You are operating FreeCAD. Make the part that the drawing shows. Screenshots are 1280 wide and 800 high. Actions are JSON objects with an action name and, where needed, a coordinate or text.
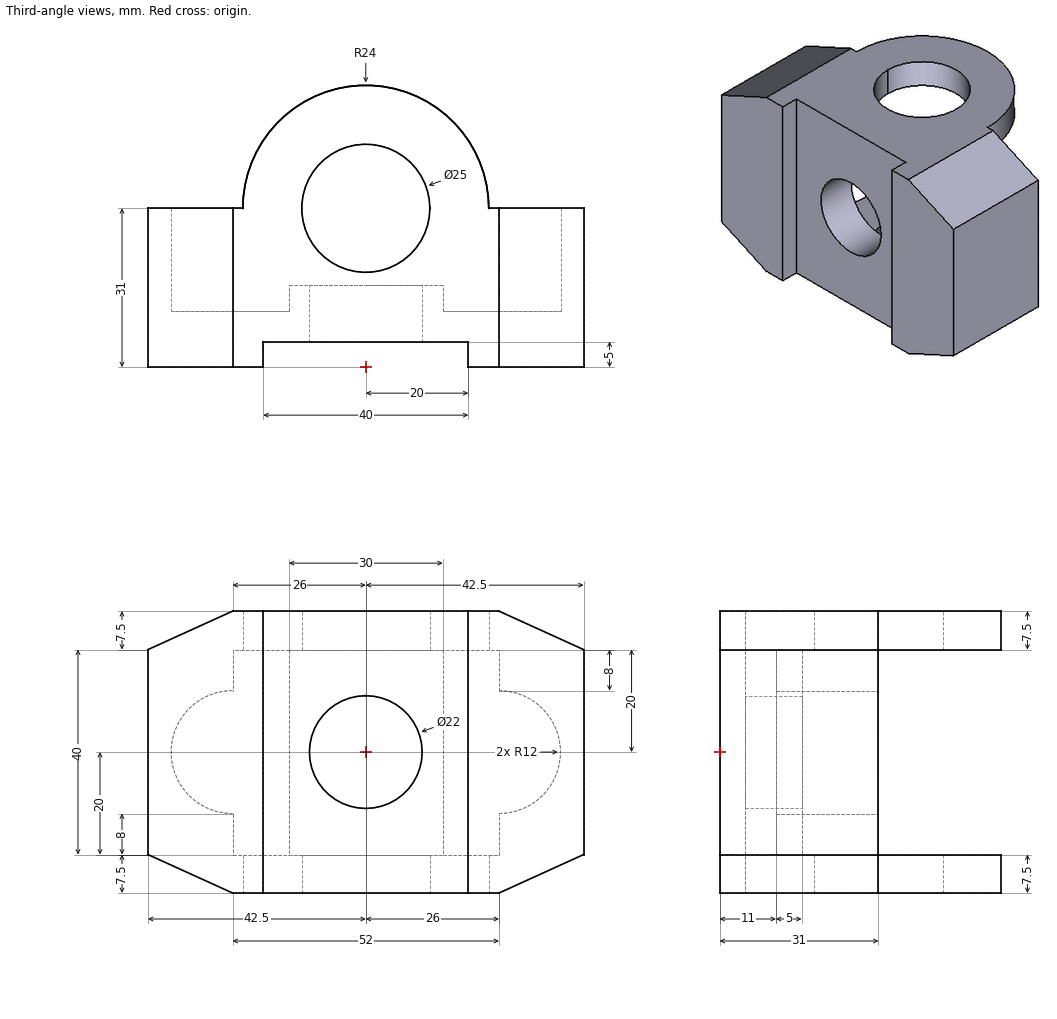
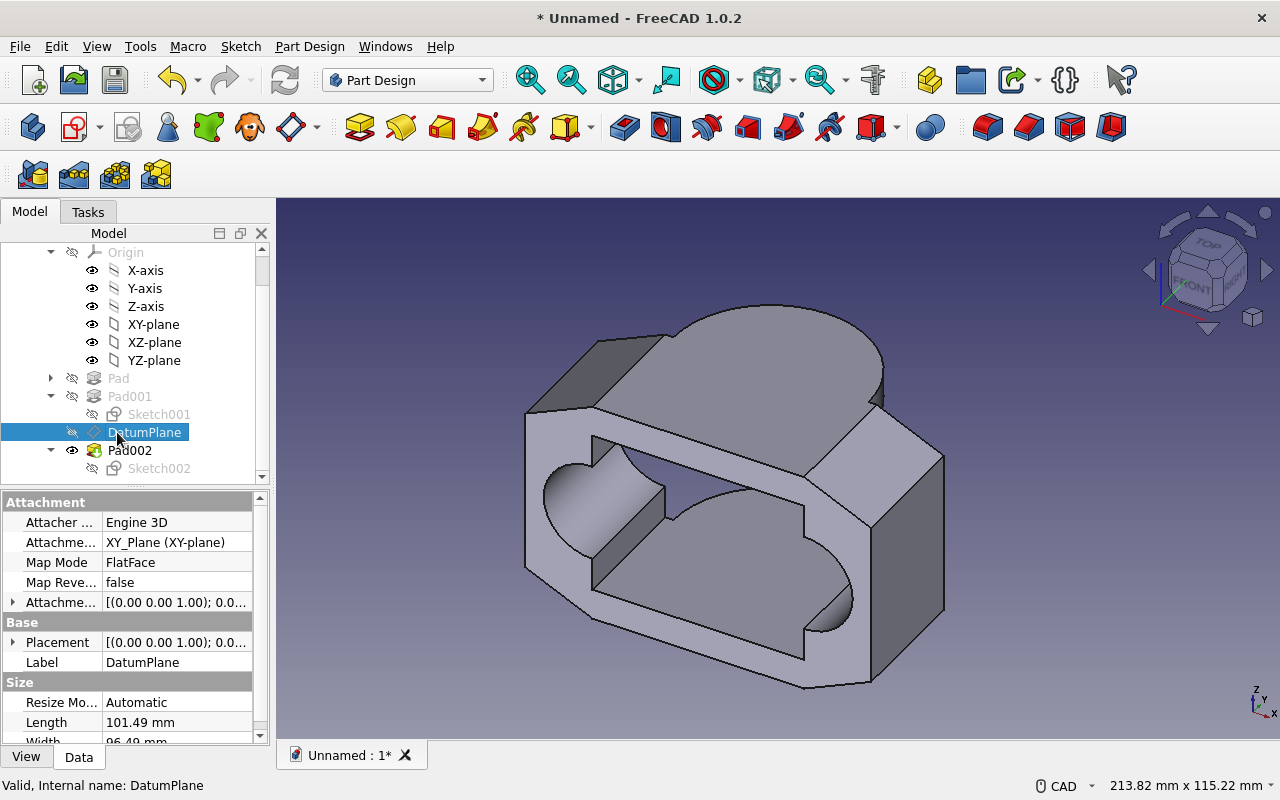
{"action": "left_click", "coordinate": [763, 377]}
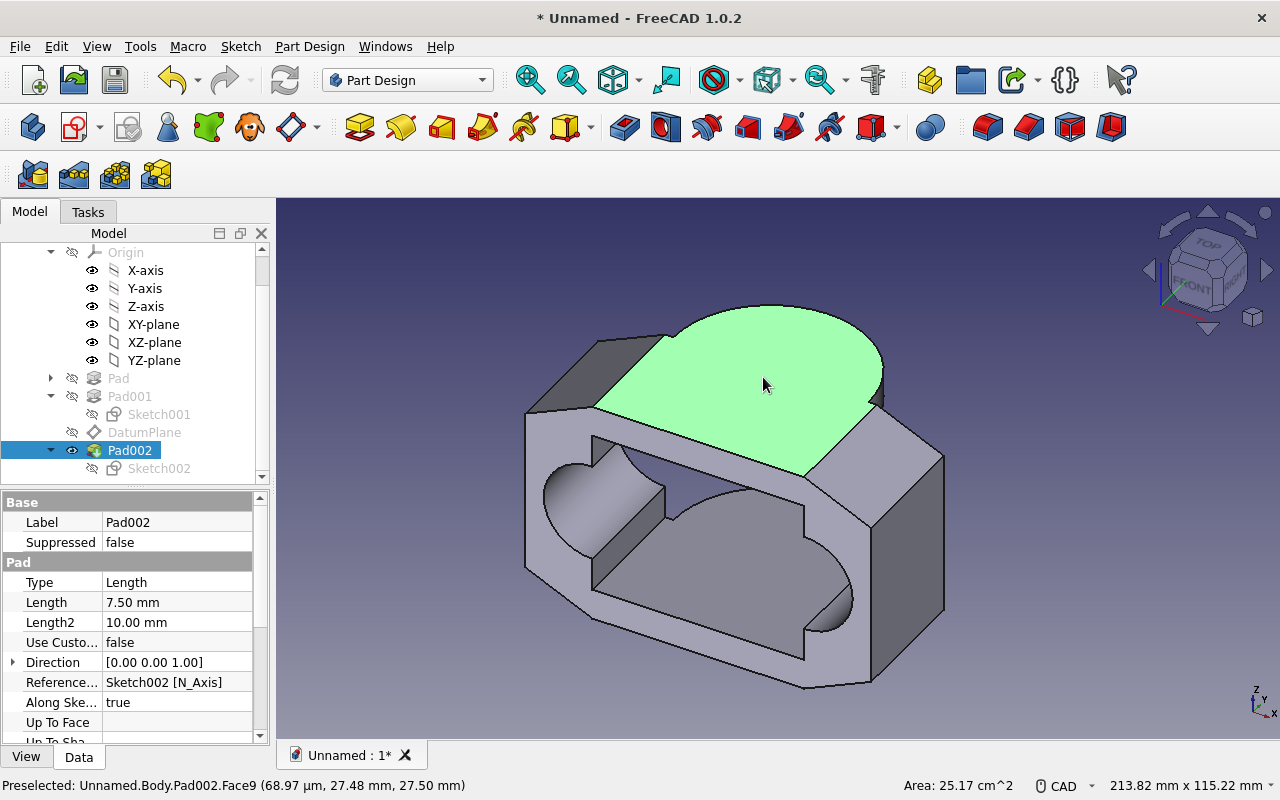
{"action": "left_click", "coordinate": [74, 128]}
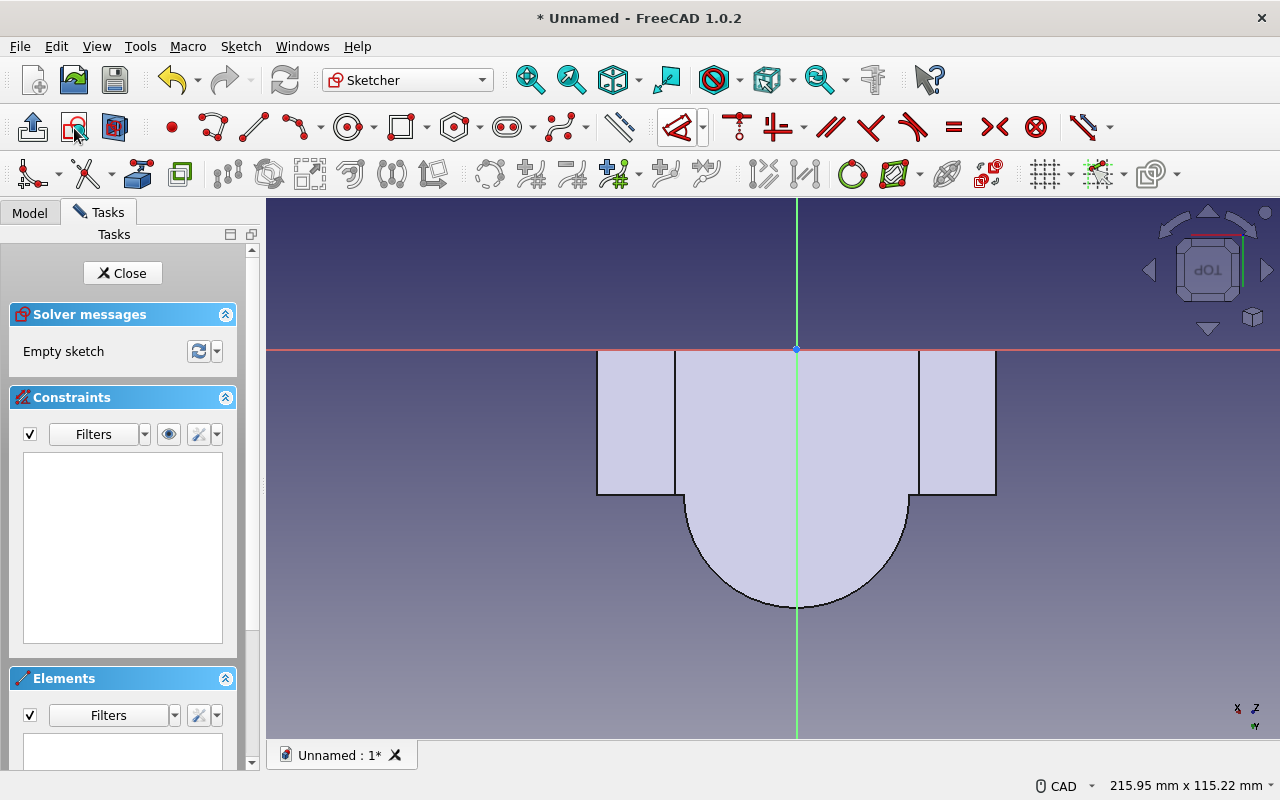
{"action": "scroll", "coordinate": [909, 432], "scroll_direction": "up", "scroll_amount": 3}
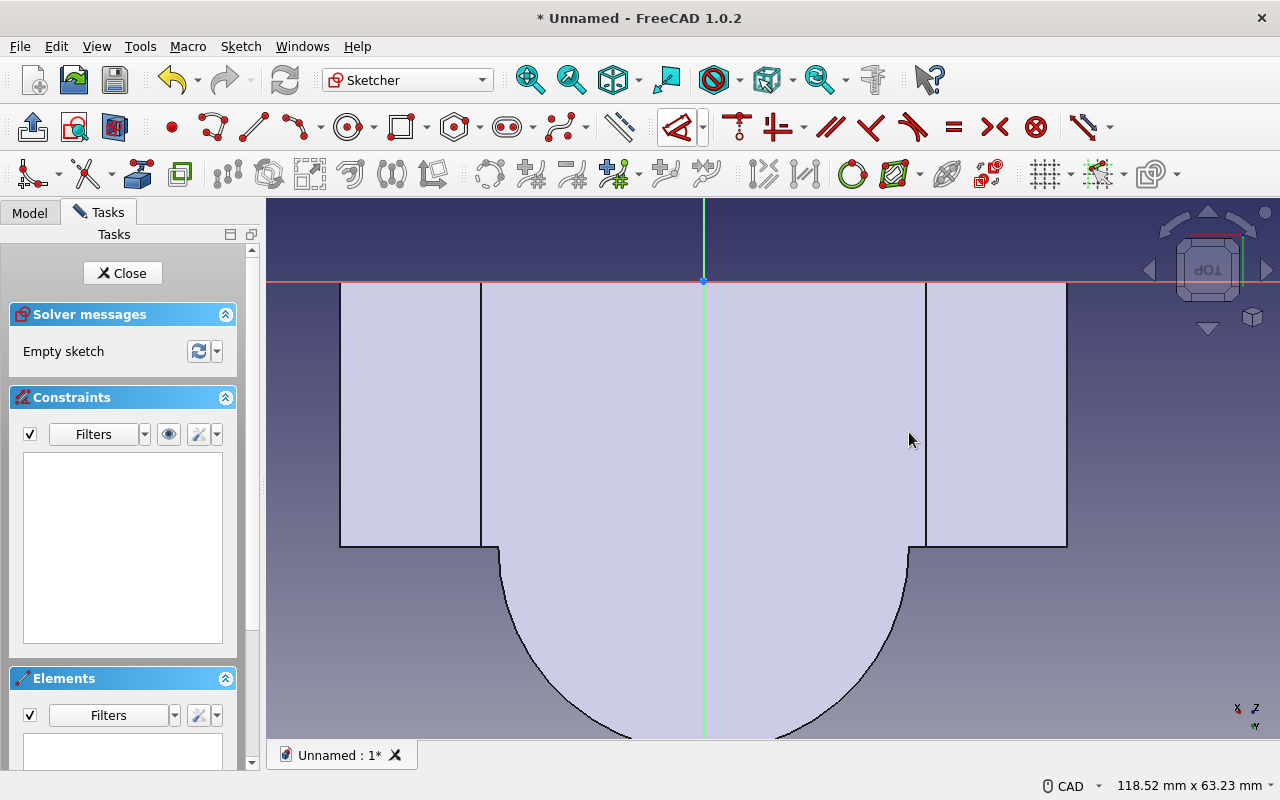
{"action": "left_click", "coordinate": [348, 128]}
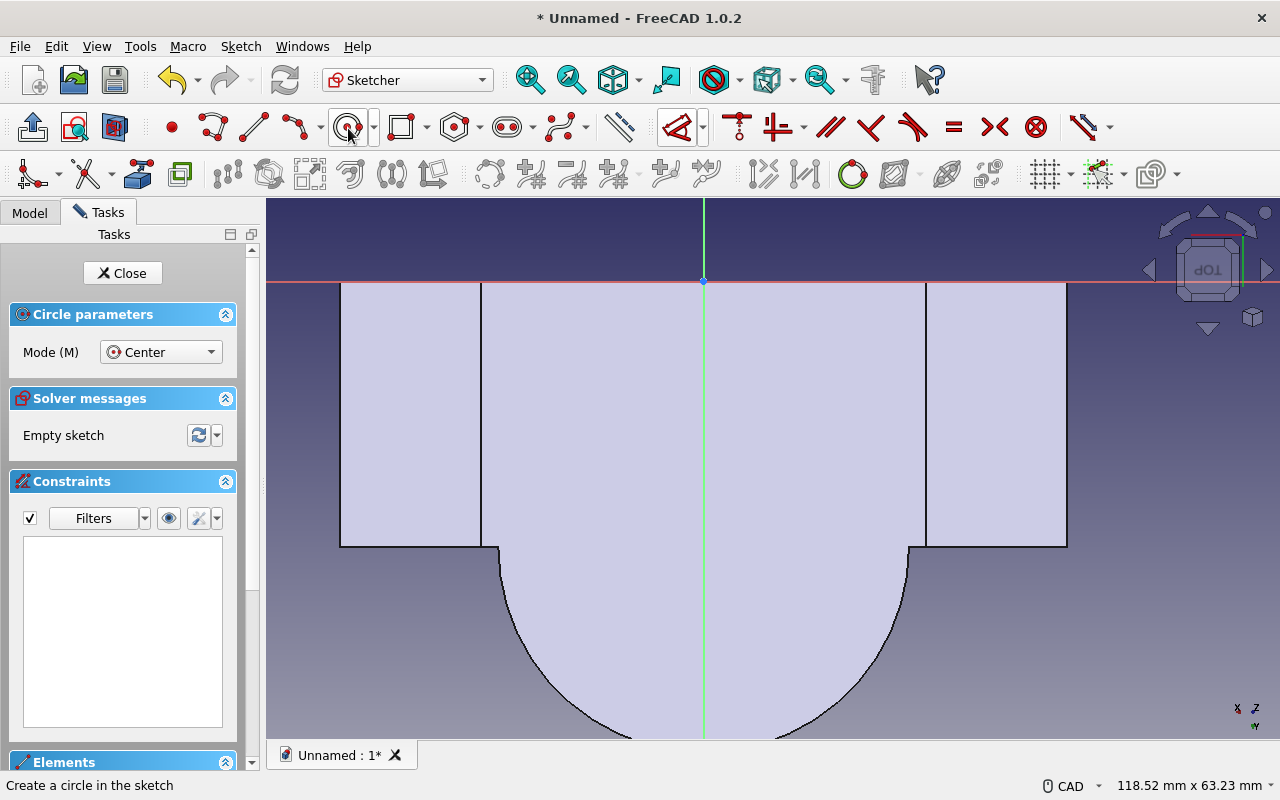
{"action": "left_click", "coordinate": [704, 547]}
{"action": "left_click", "coordinate": [779, 471]}
{"action": "key", "text": "Escape"}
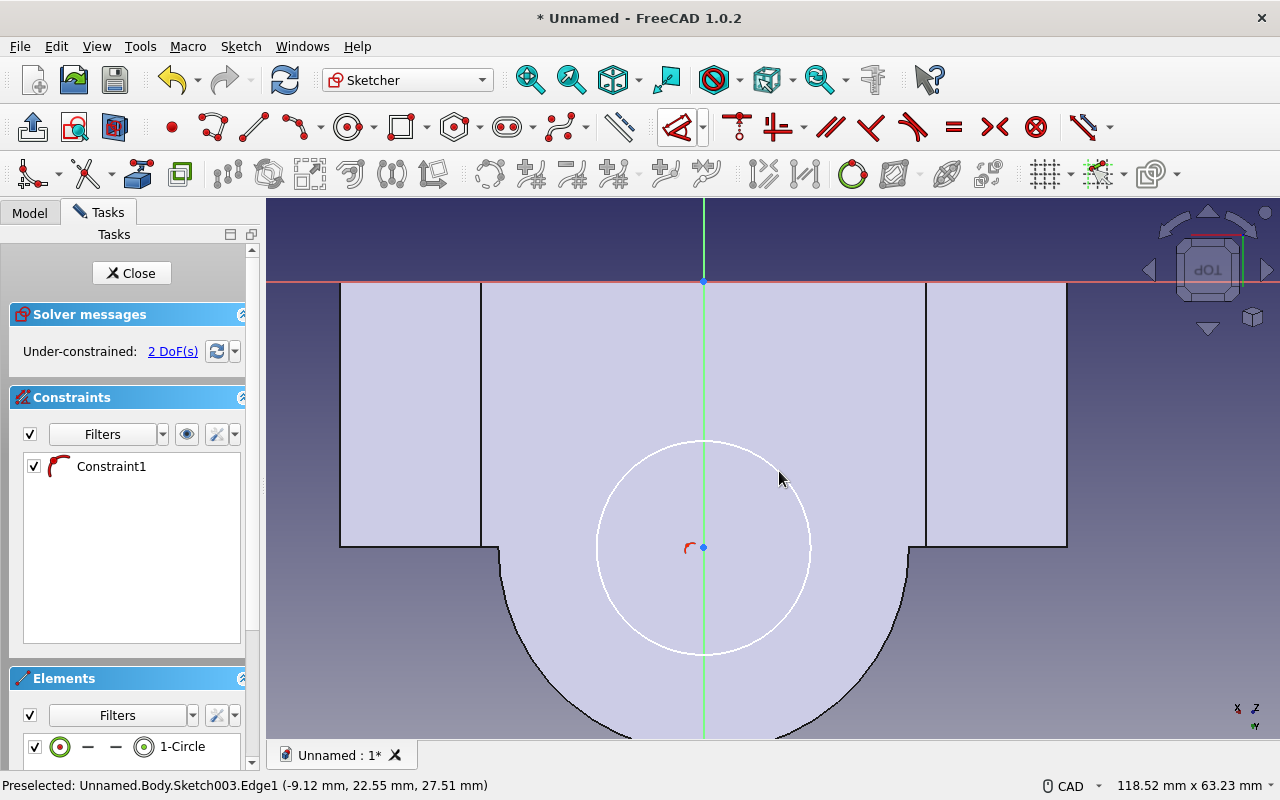
{"action": "left_click", "coordinate": [779, 472]}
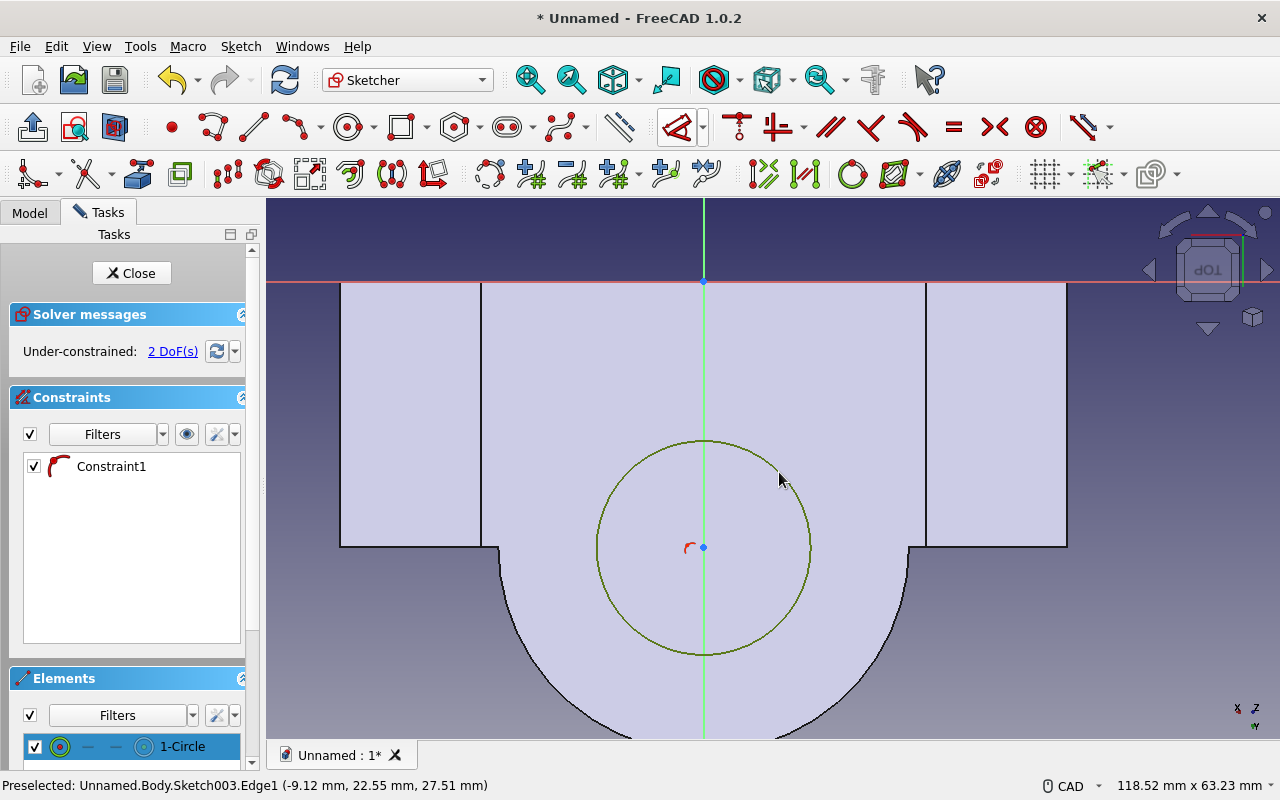
{"action": "key", "text": "k o"}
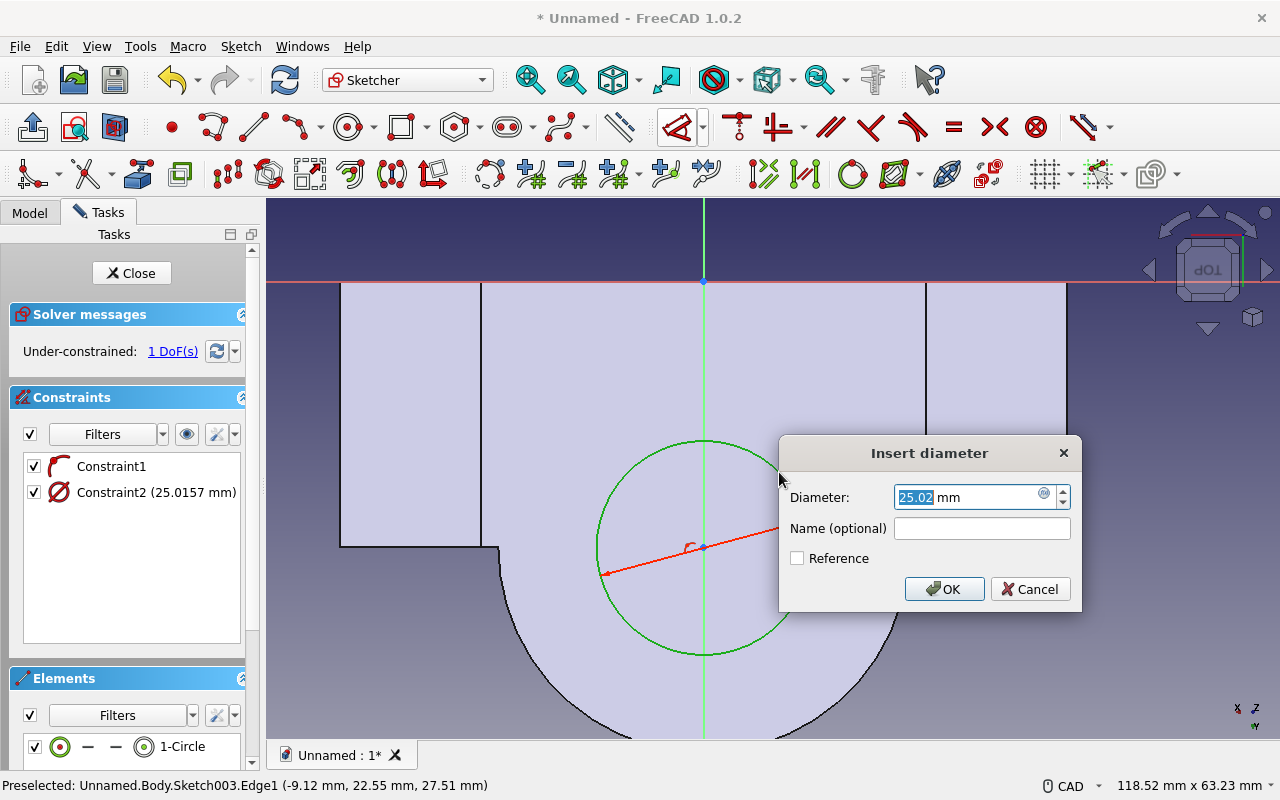
{"action": "type", "text": "25"}
{"action": "key", "text": "Return"}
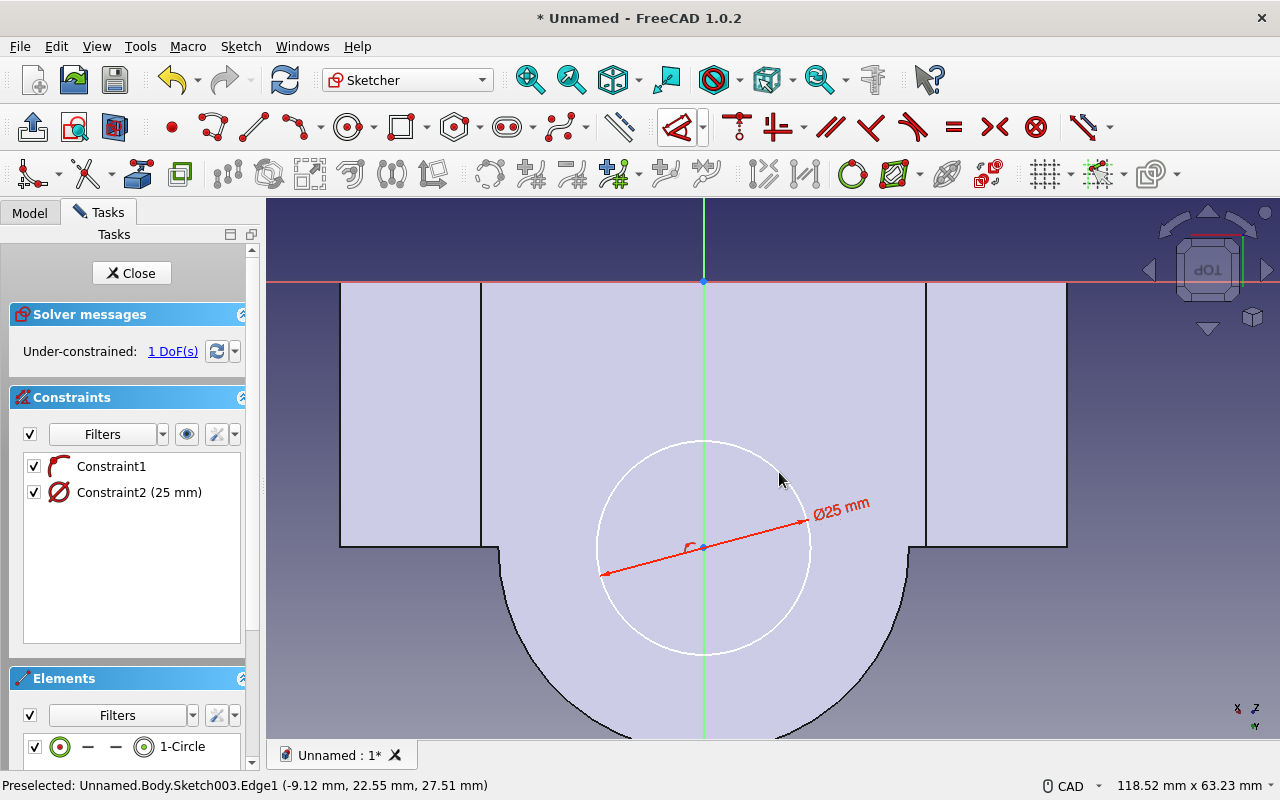
{"action": "left_click", "coordinate": [704, 548]}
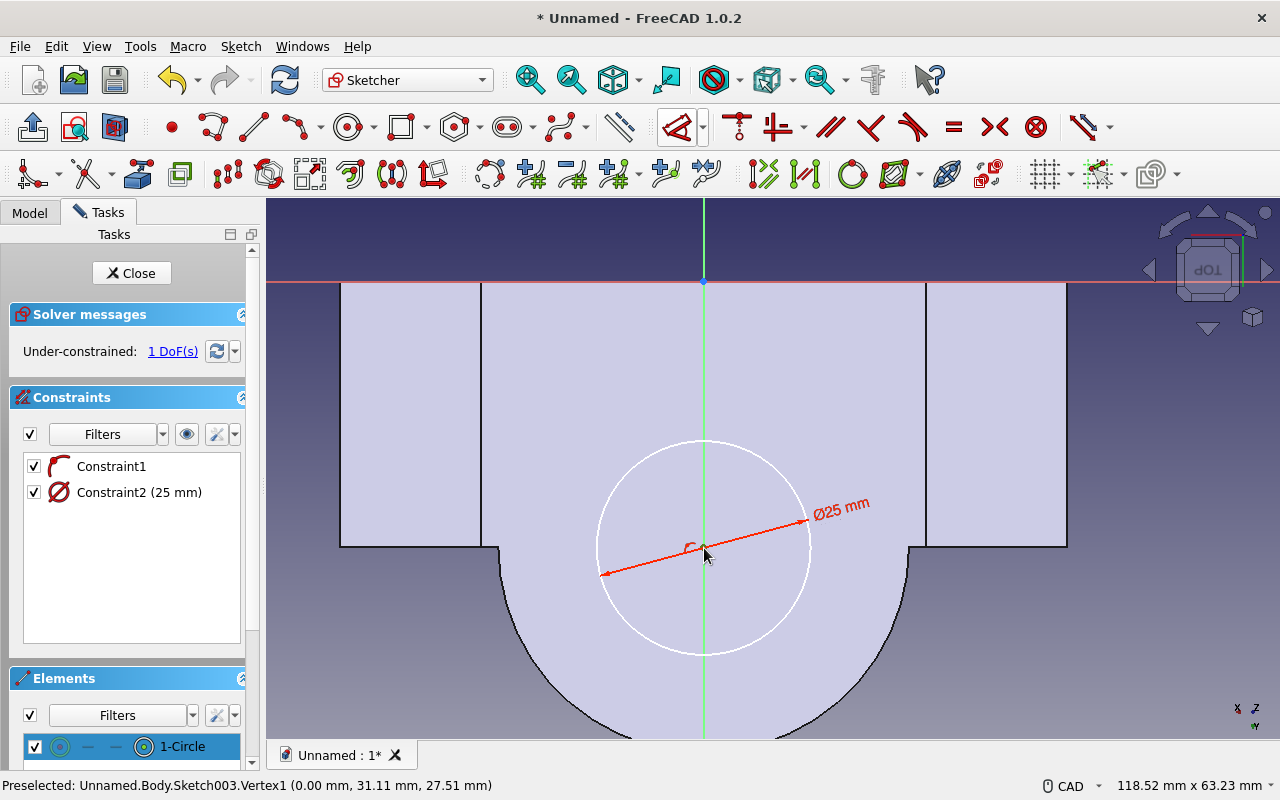
{"action": "left_click", "coordinate": [702, 128]}